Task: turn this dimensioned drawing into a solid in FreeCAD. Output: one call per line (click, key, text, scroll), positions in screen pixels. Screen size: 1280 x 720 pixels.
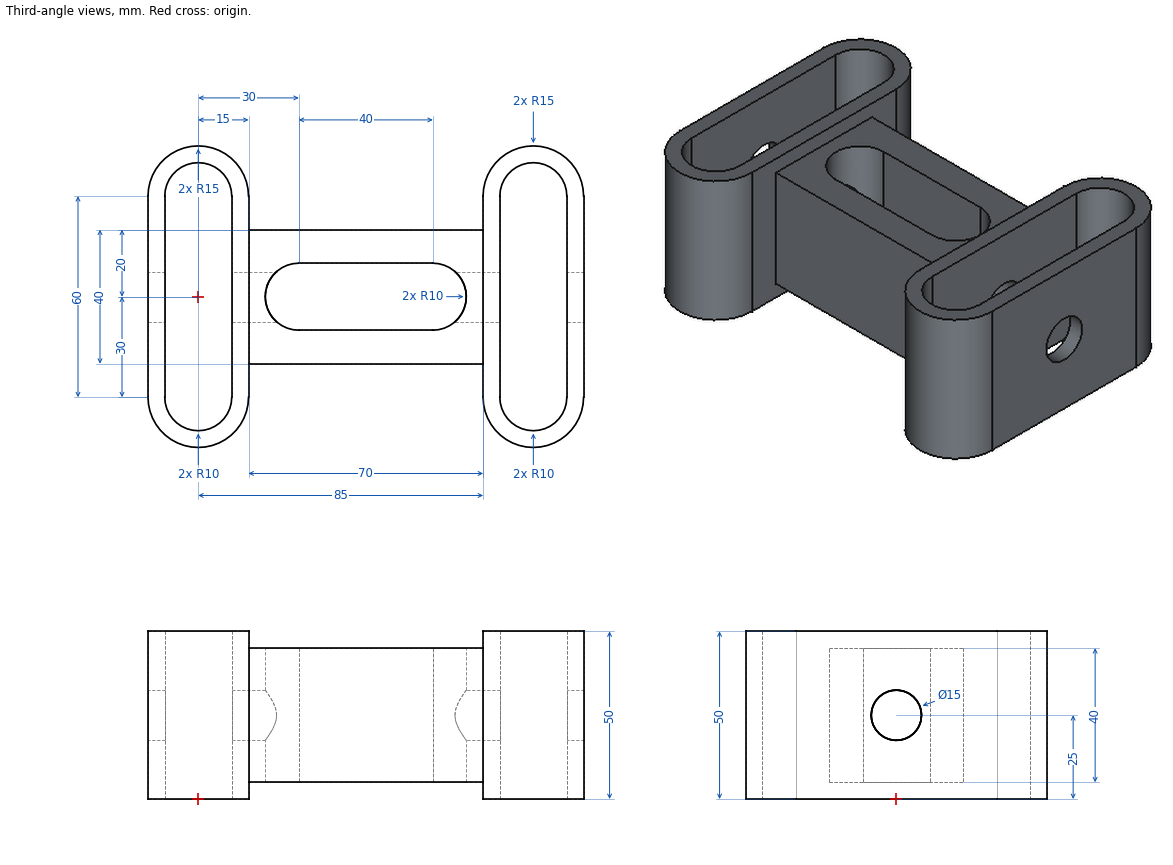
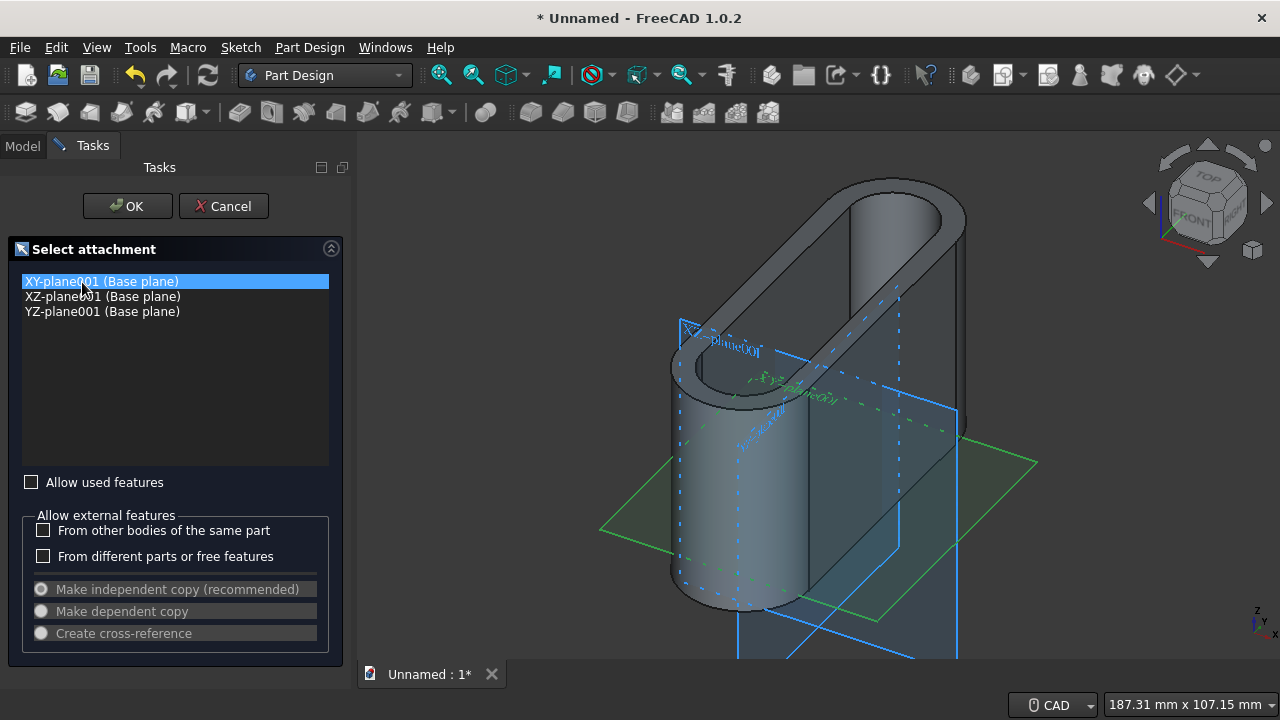
click(128, 206)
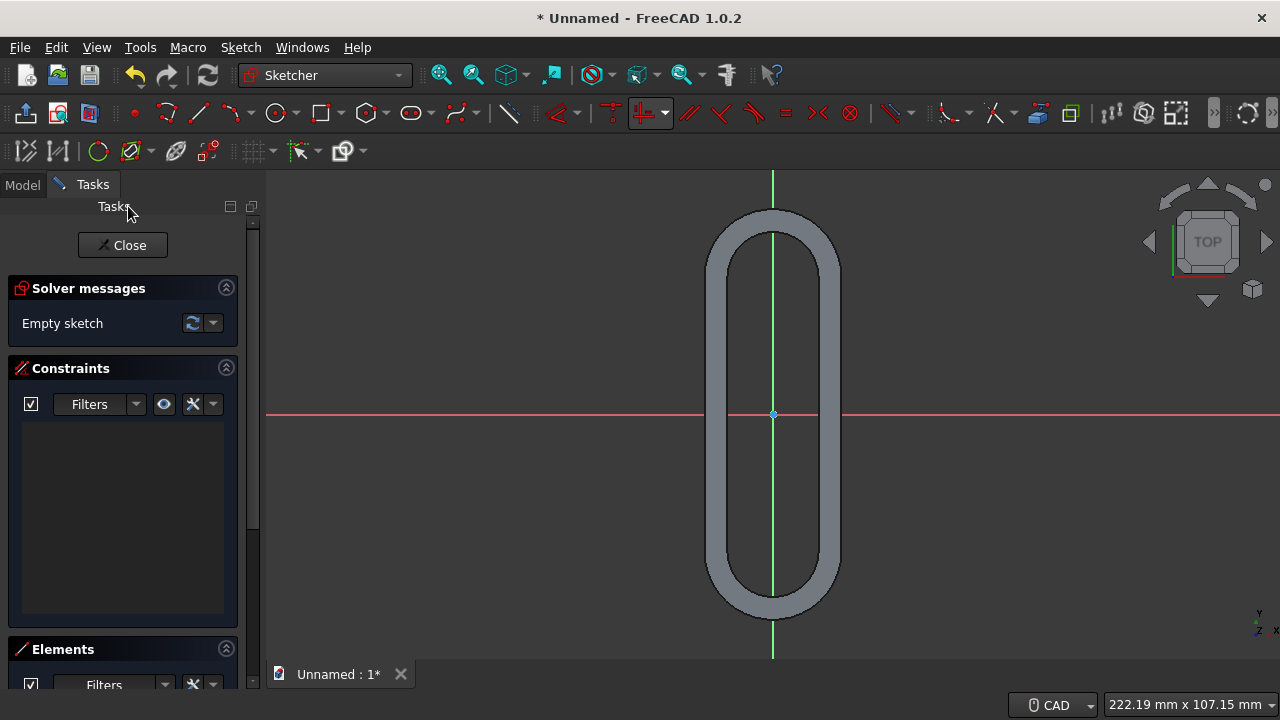
scroll(294, 414, down, 2)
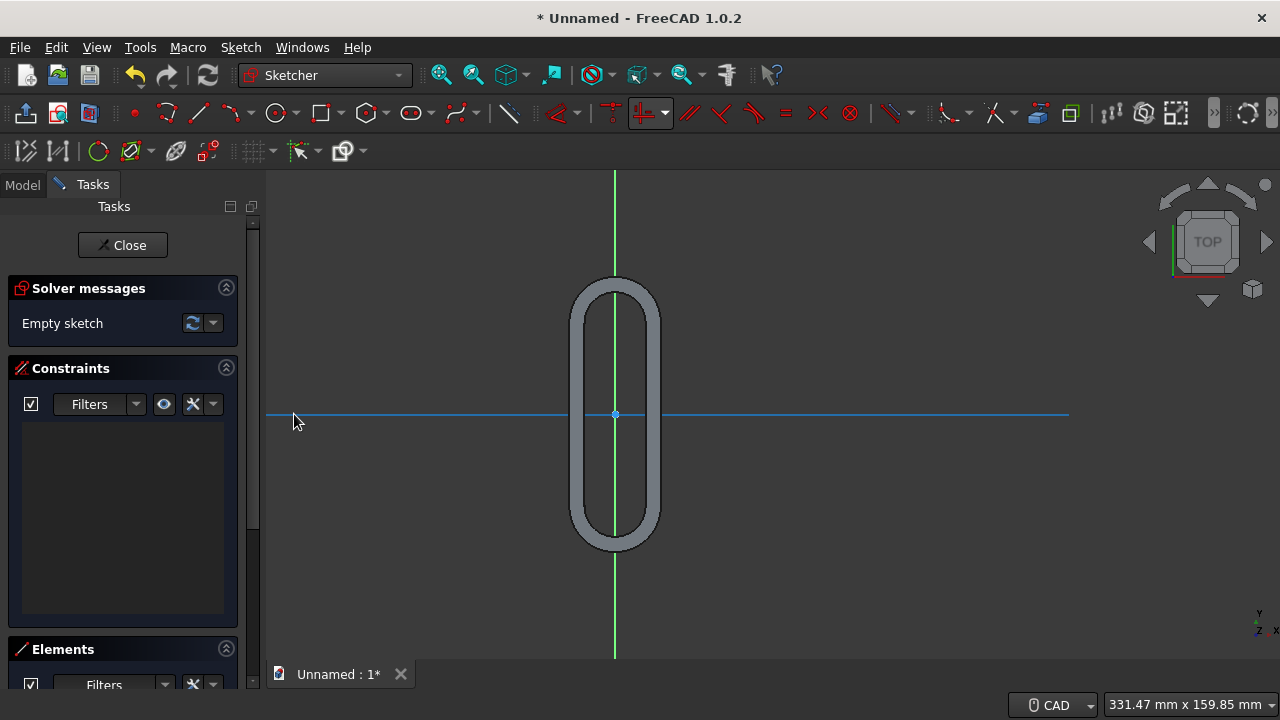
click(412, 114)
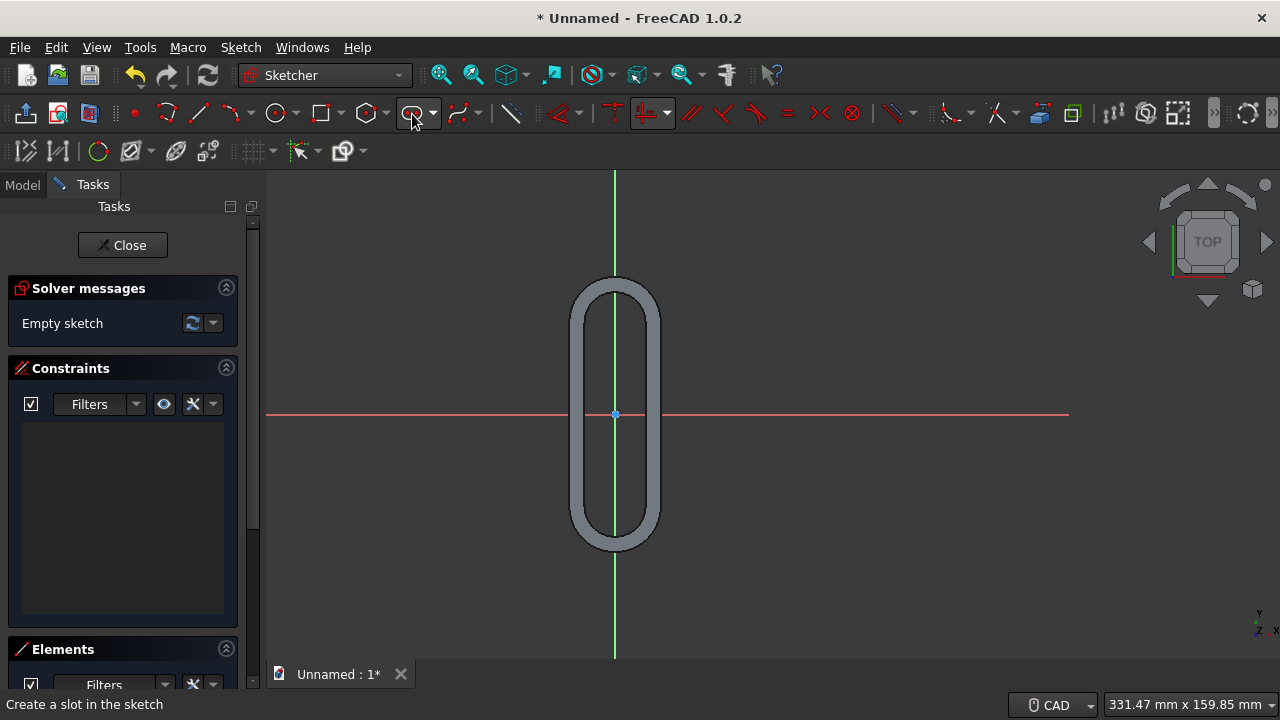
click(921, 506)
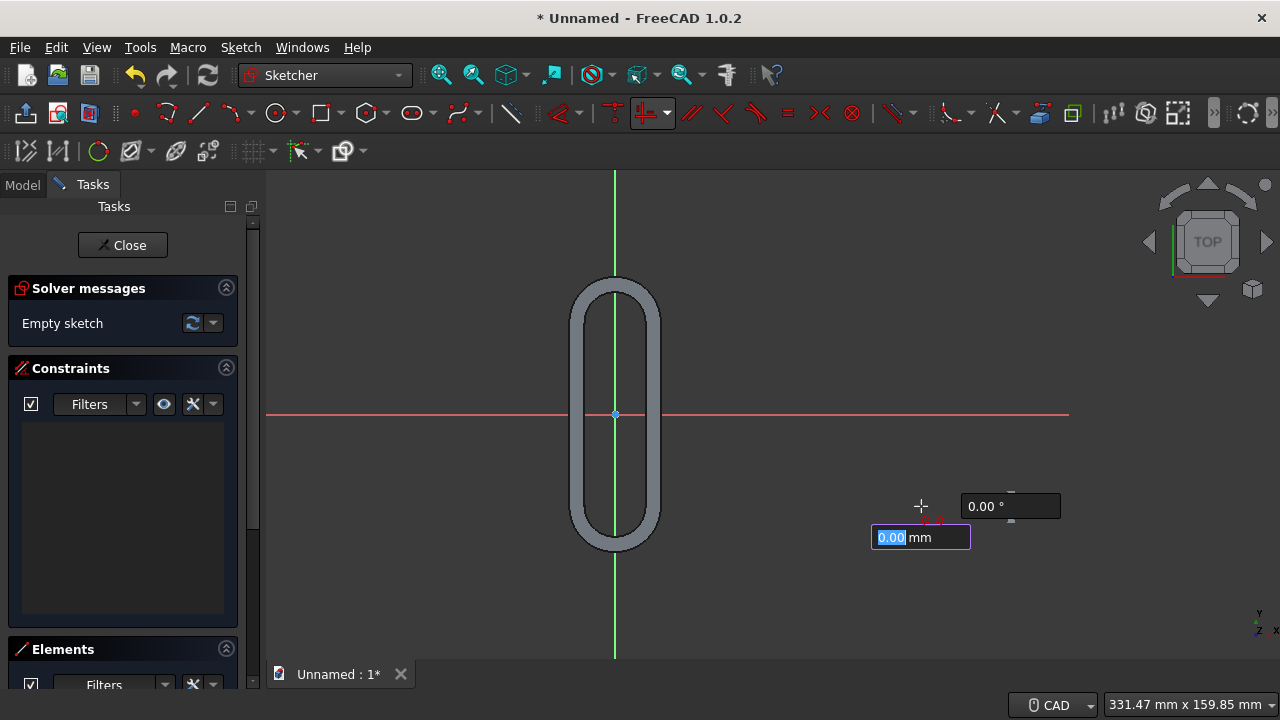
click(921, 323)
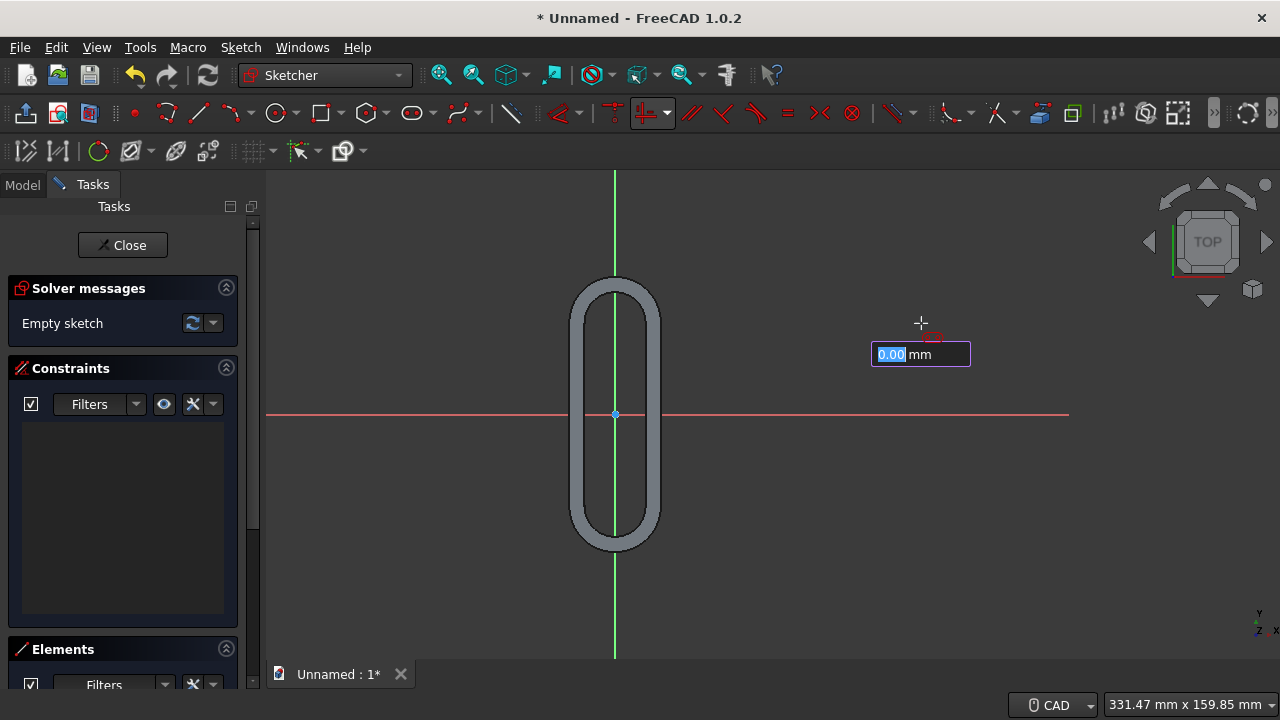
click(967, 442)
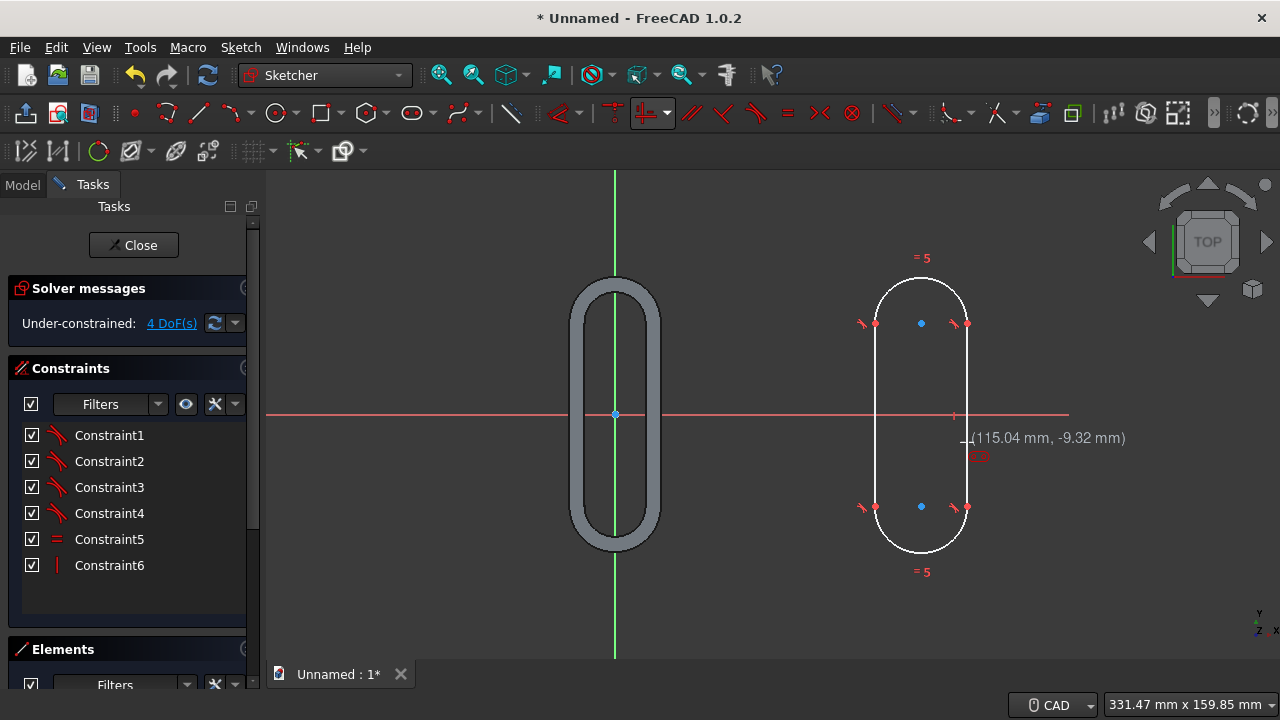
click(921, 507)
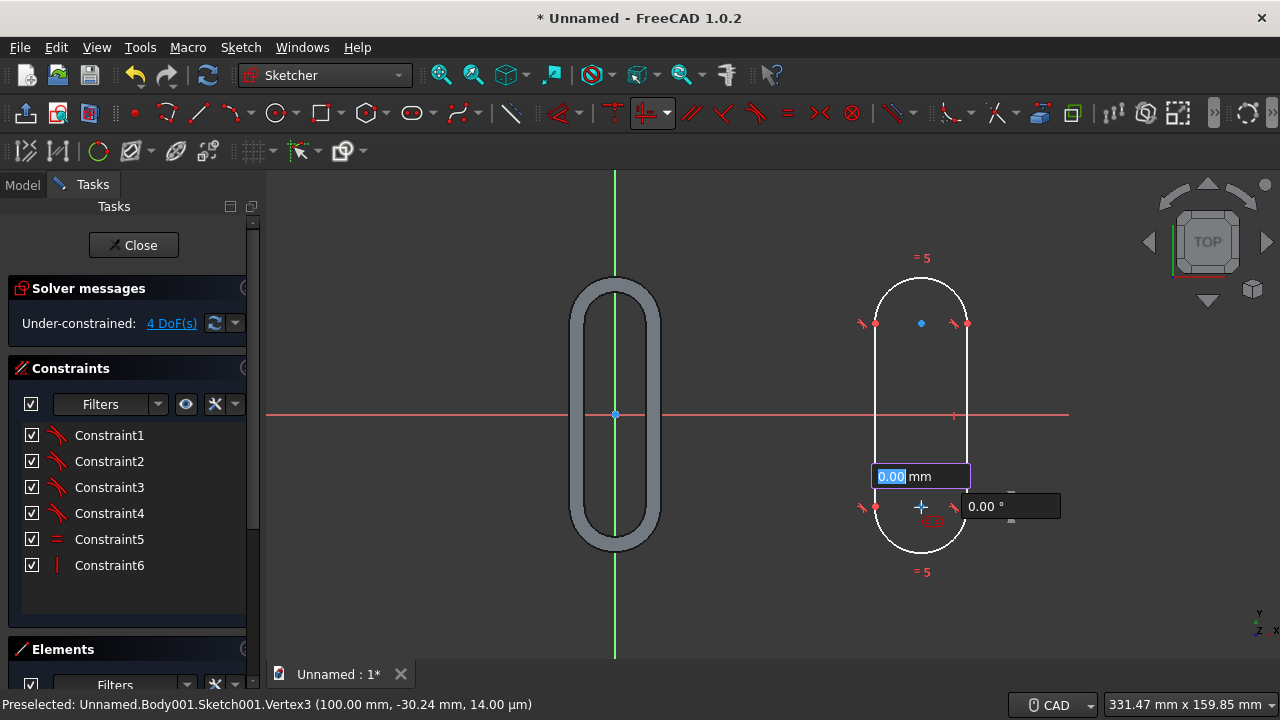
click(921, 324)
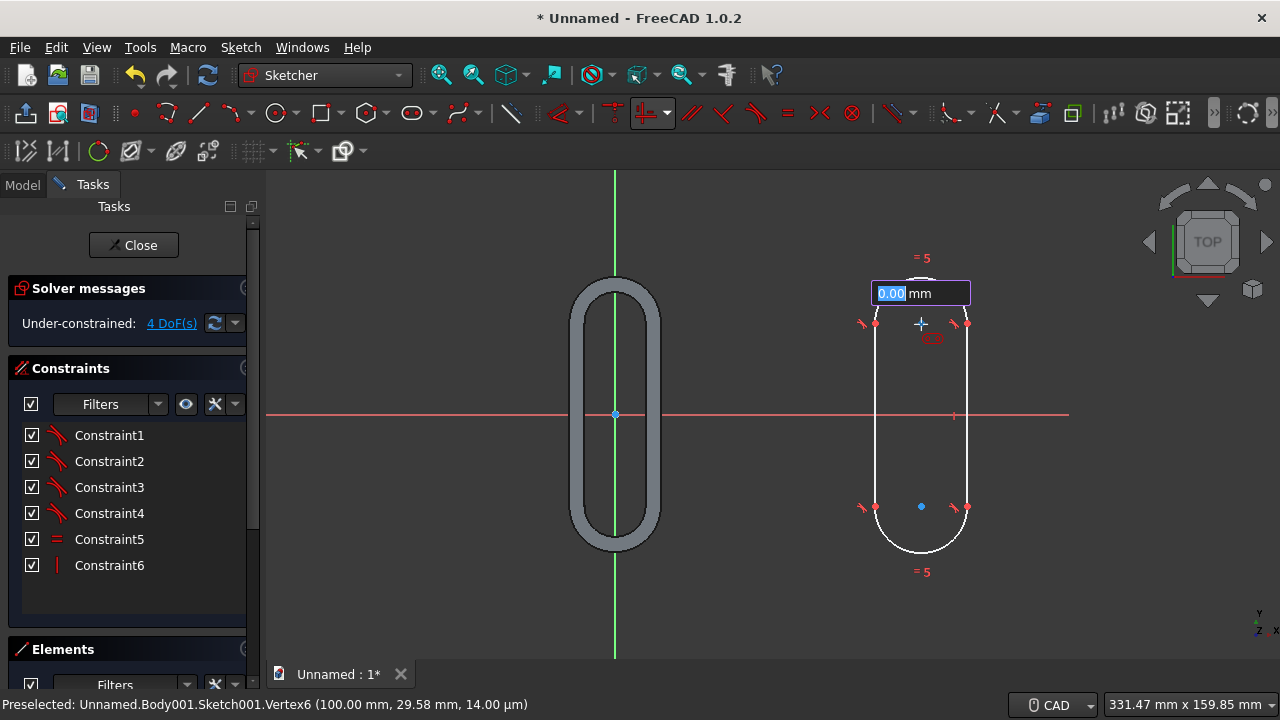
click(952, 387)
key(Escape)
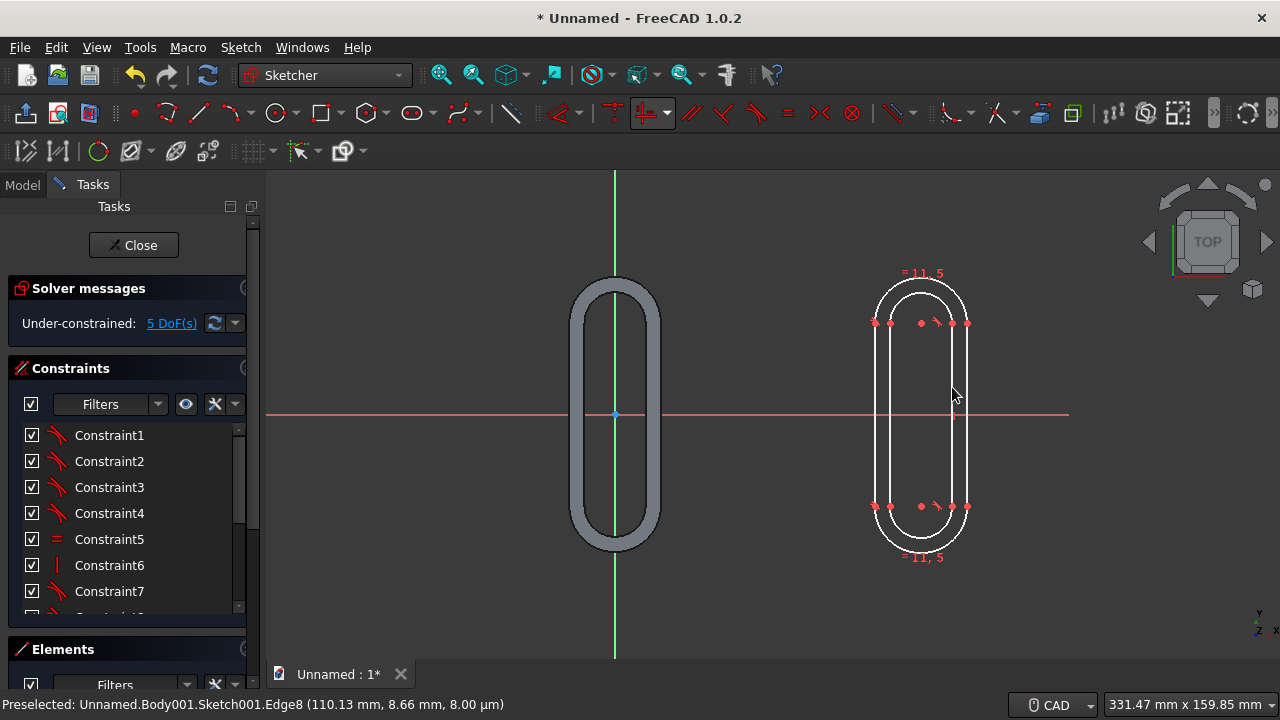
click(558, 114)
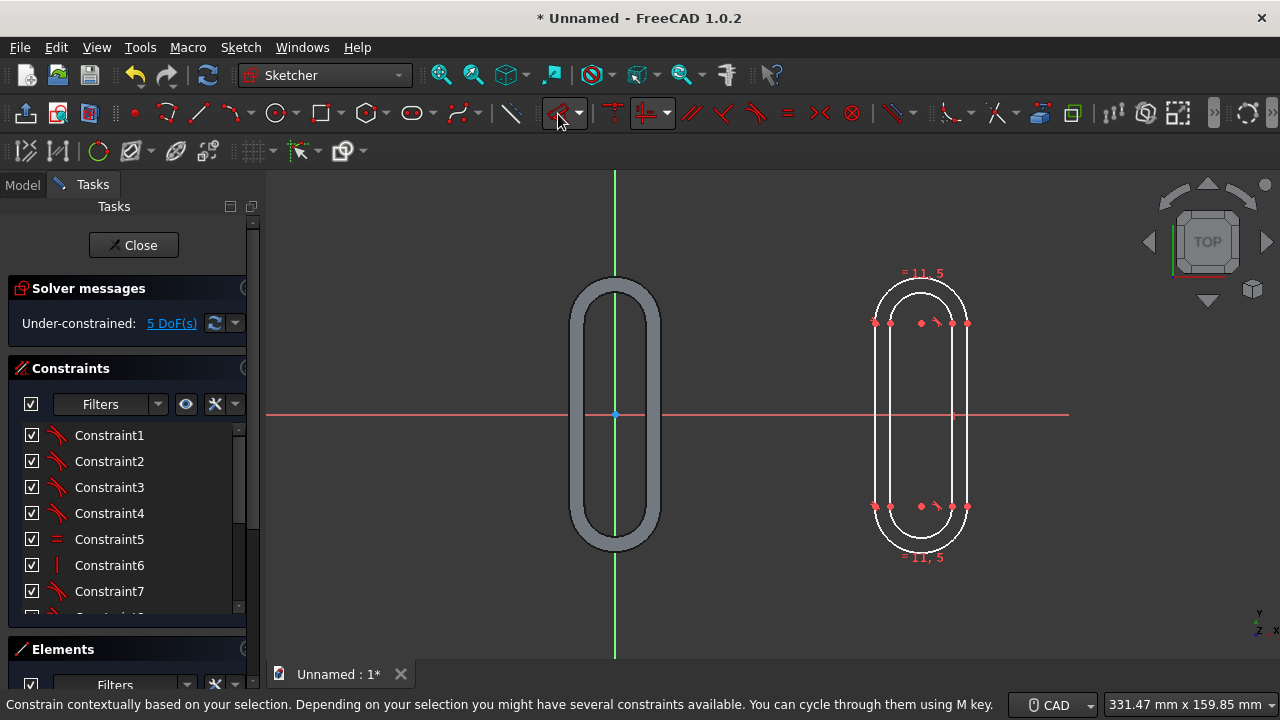
click(894, 544)
click(875, 570)